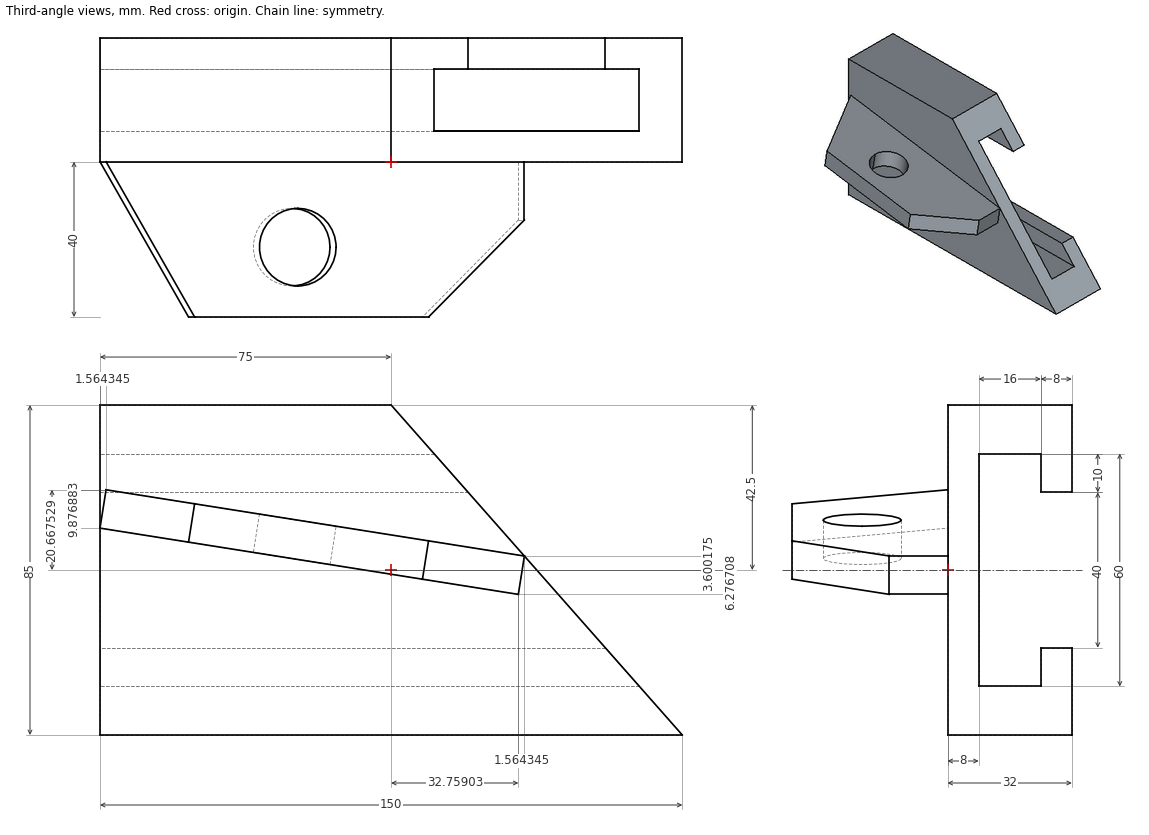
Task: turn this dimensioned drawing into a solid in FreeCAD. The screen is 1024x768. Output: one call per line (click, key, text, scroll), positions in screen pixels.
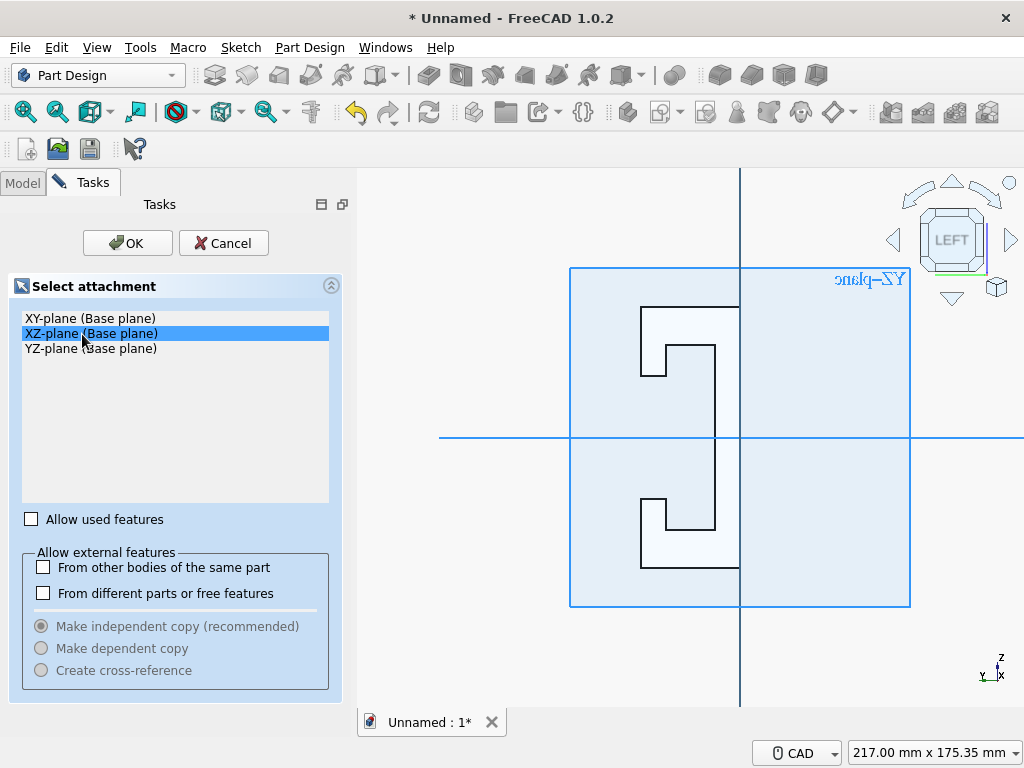
click(128, 243)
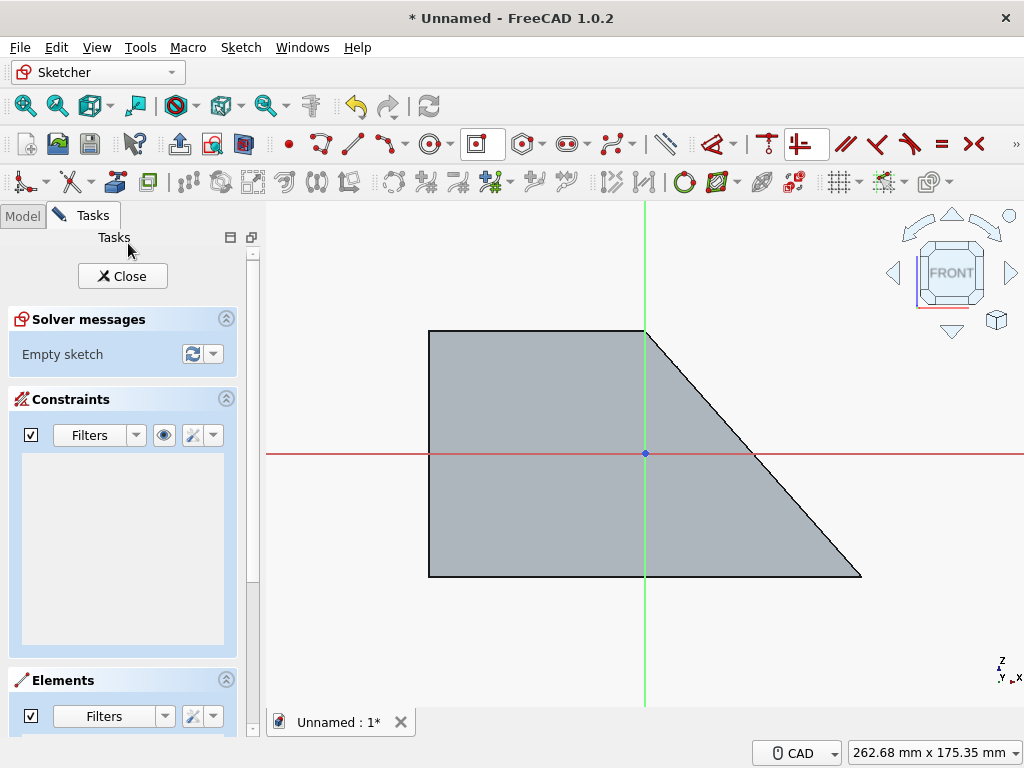
click(322, 144)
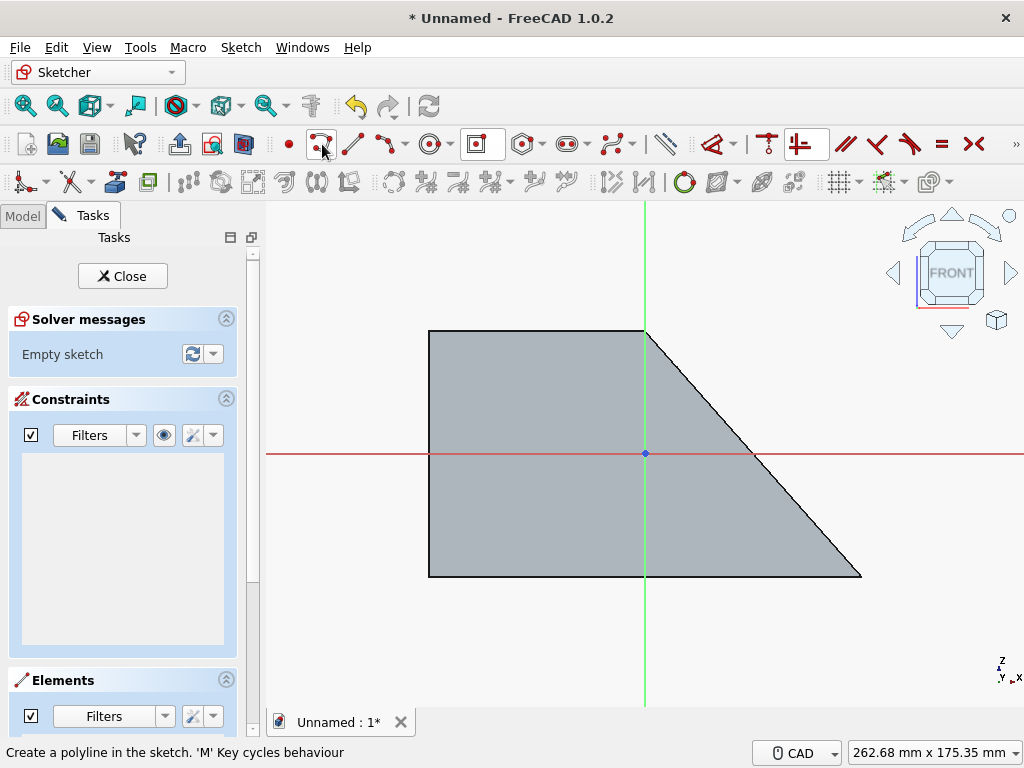
click(740, 472)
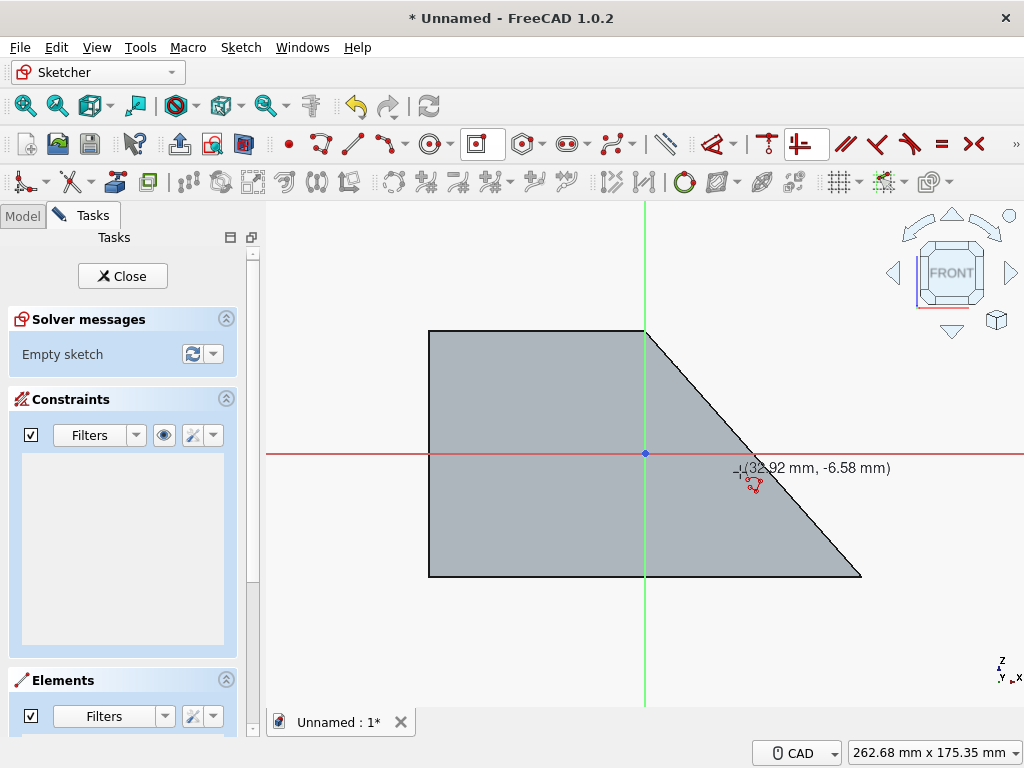
scroll(744, 444, up, 3)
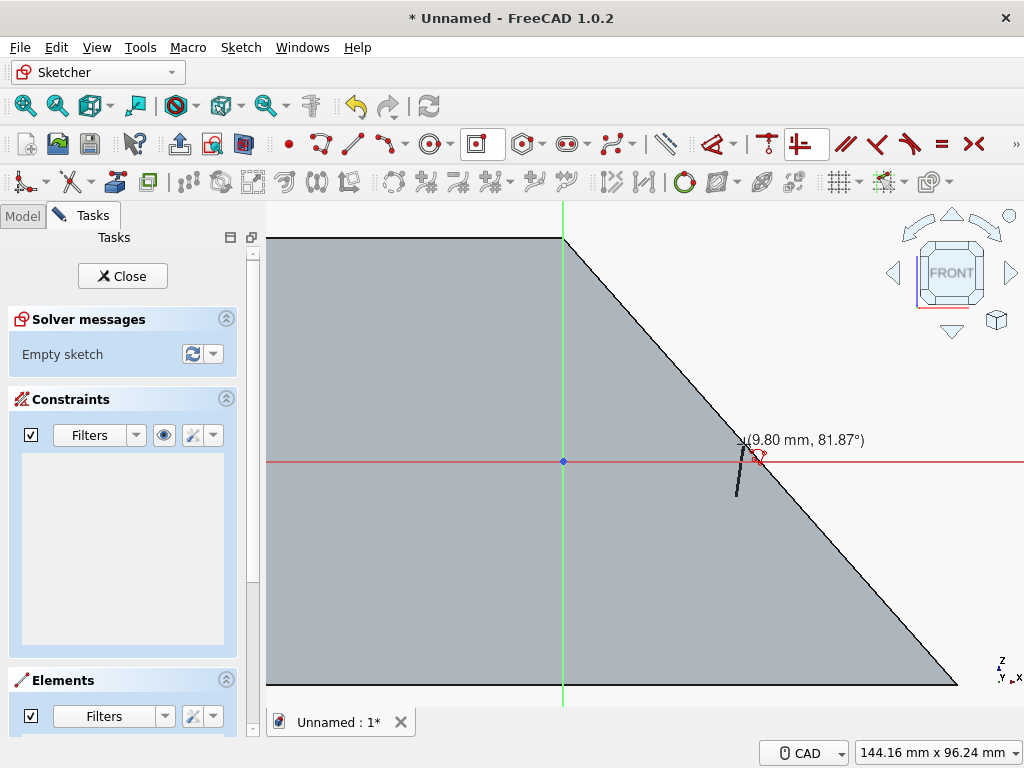
click(744, 443)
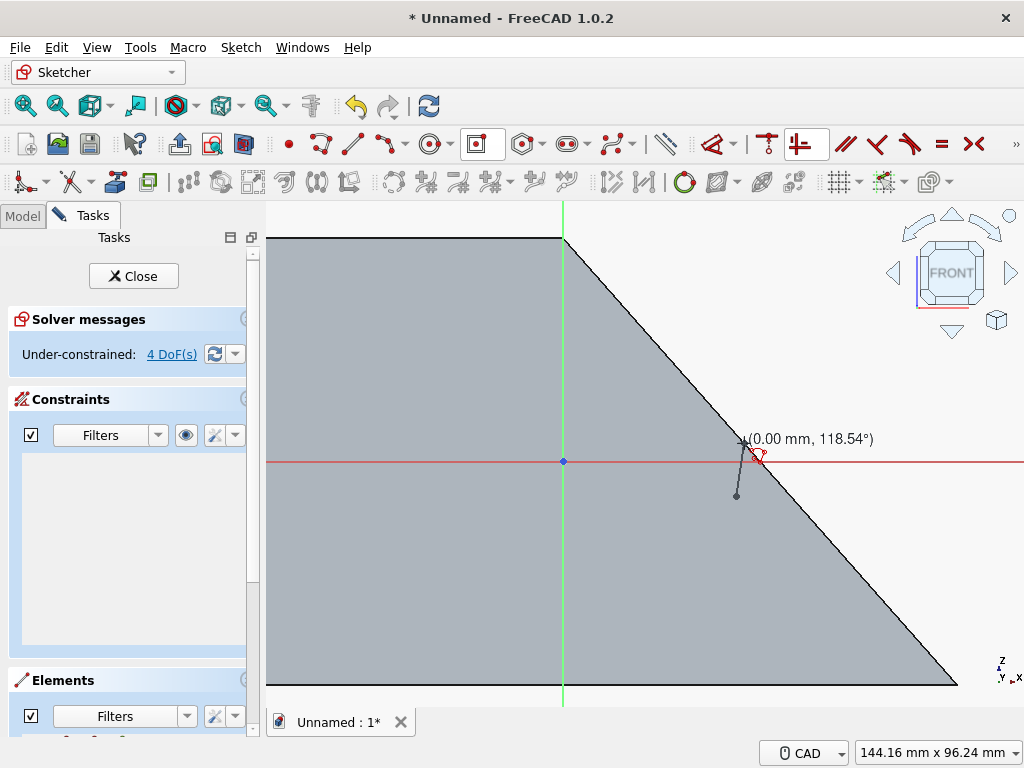
scroll(821, 515, down, 2)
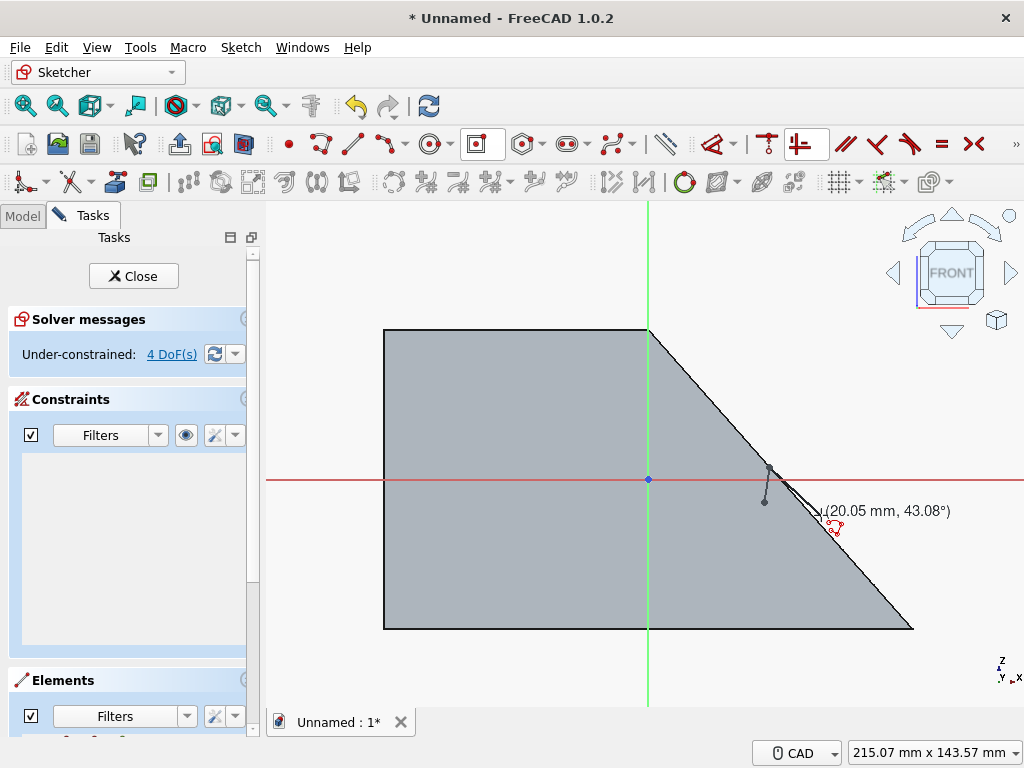
click(390, 407)
click(384, 442)
click(764, 503)
key(Escape)
key(Escape)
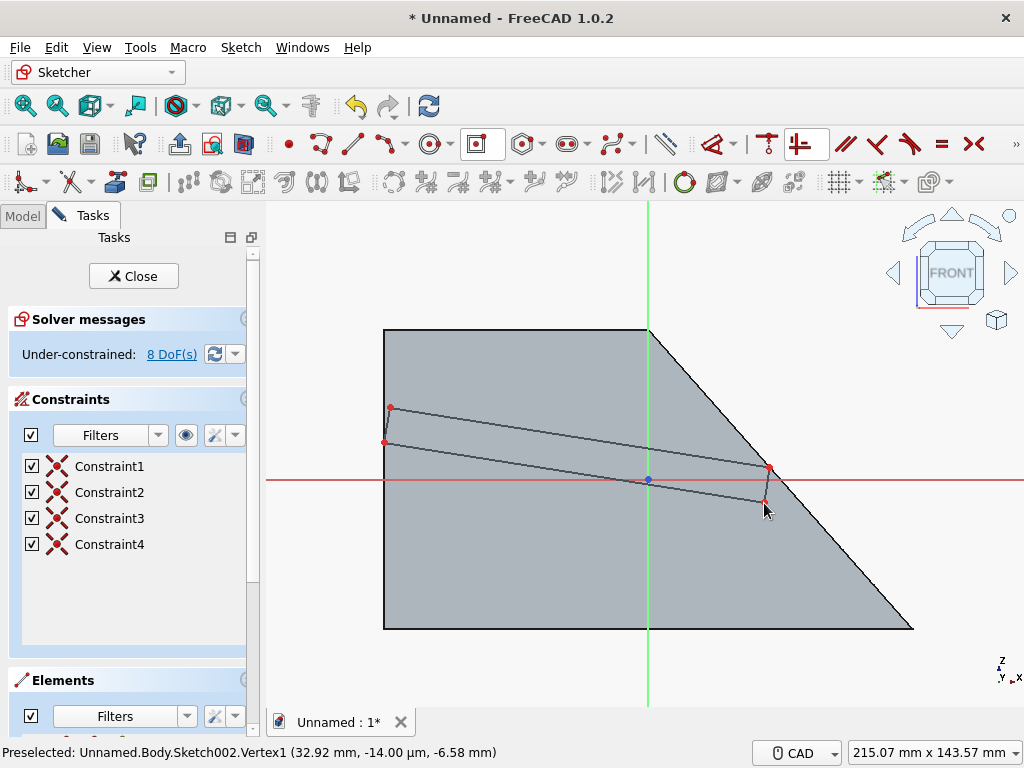
key(d)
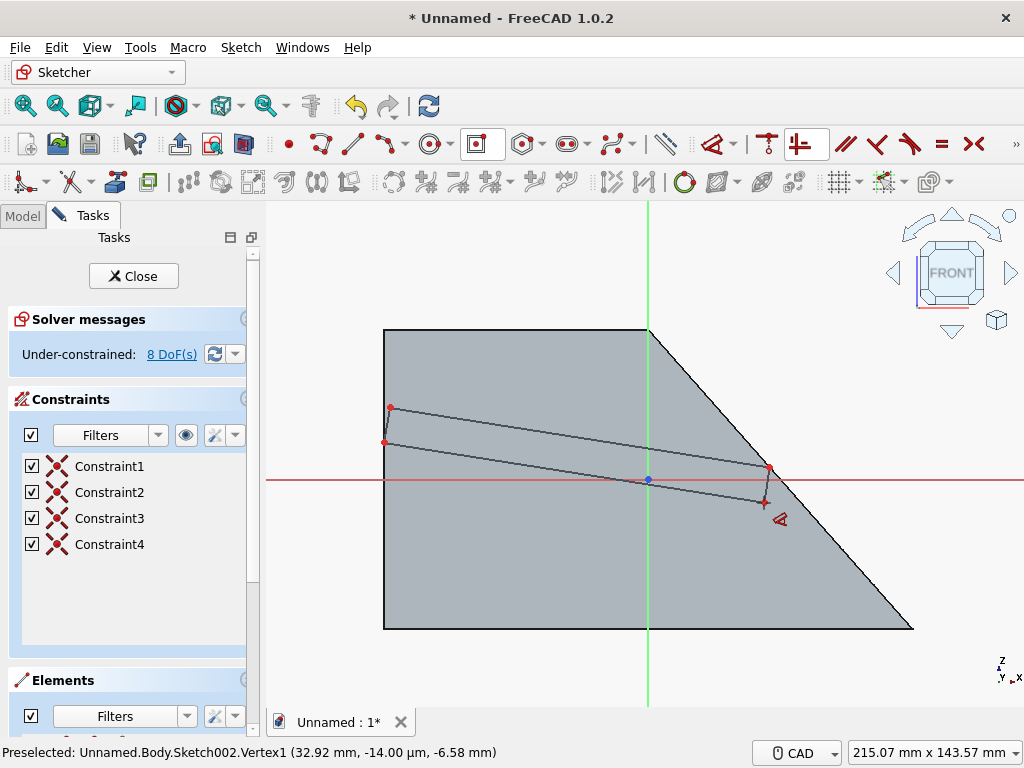
click(384, 443)
click(516, 514)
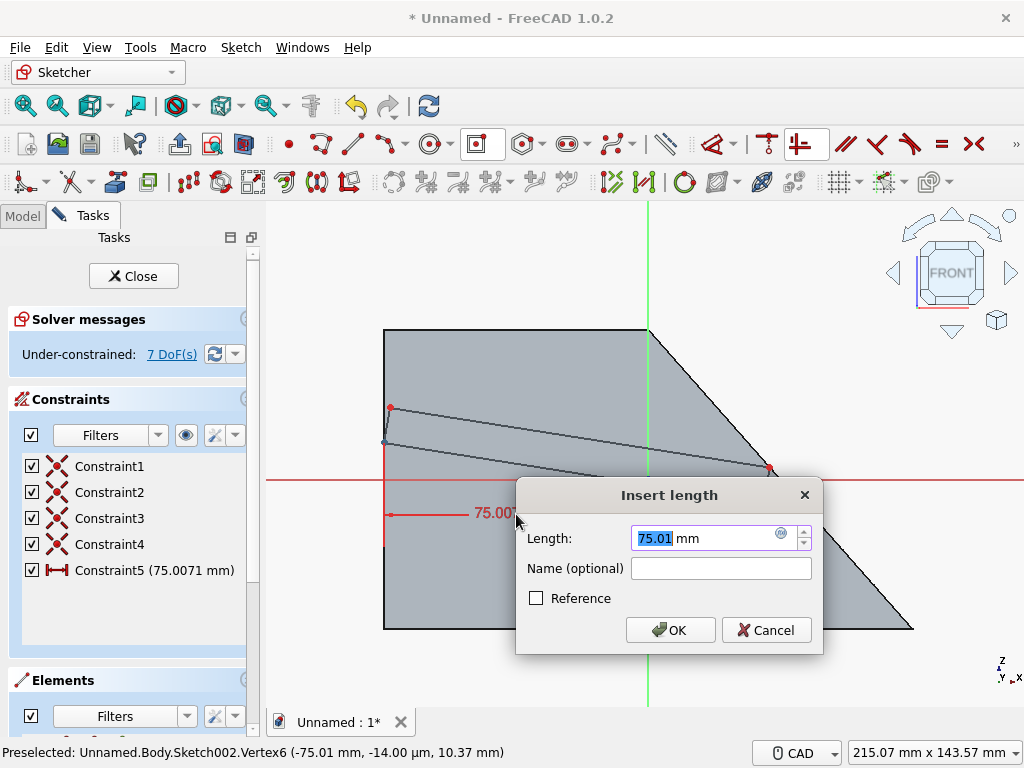
text(75)
key(Return)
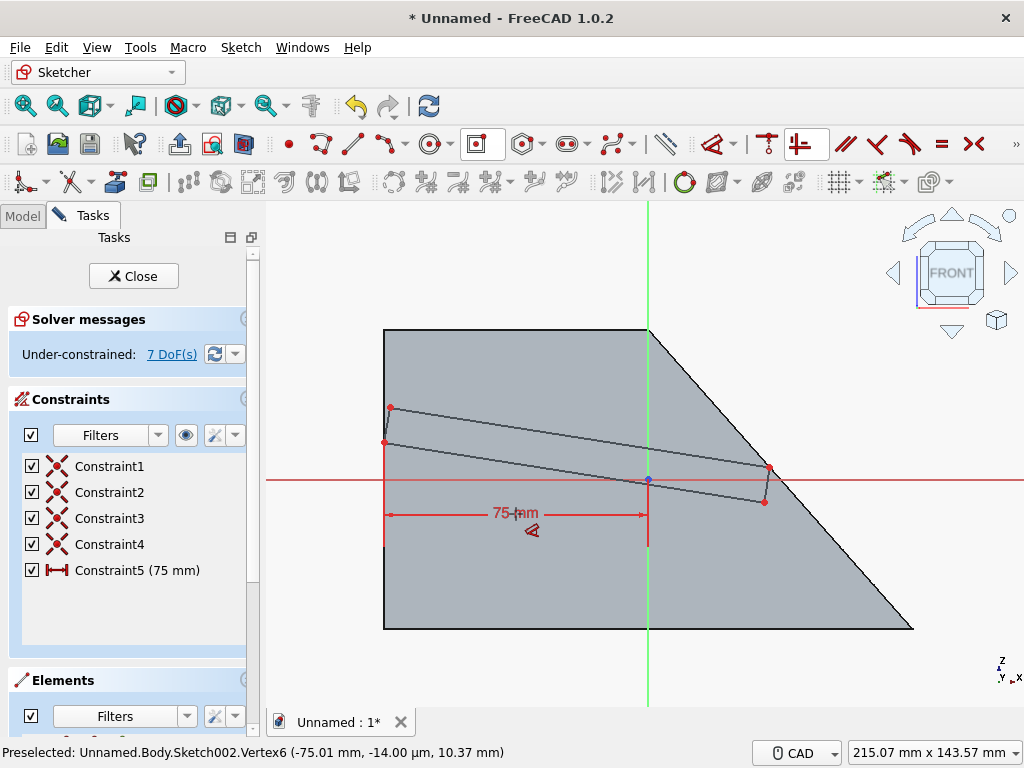
click(764, 503)
click(706, 537)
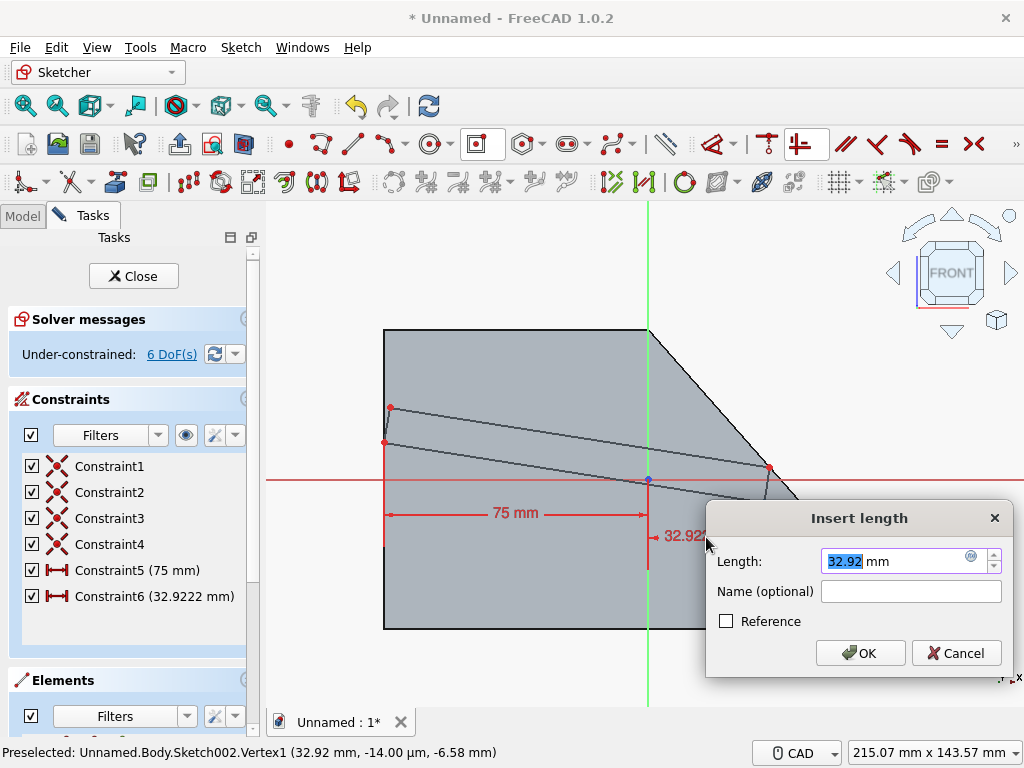
text(32.75903)
key(Return)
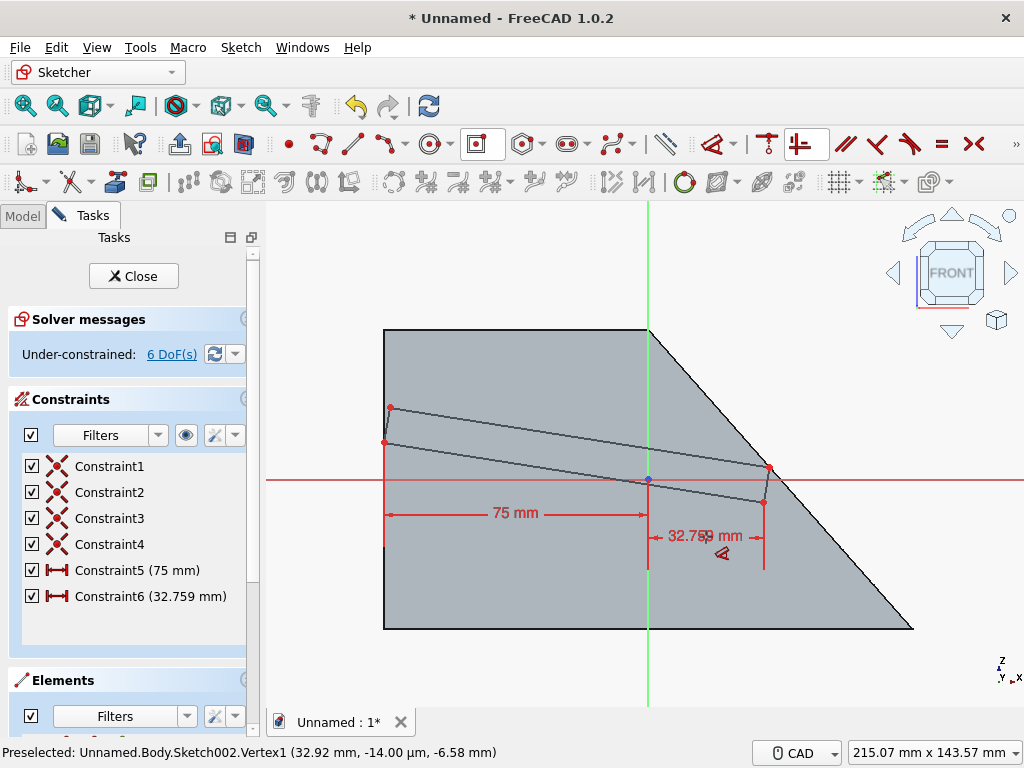
scroll(764, 503, up, 3)